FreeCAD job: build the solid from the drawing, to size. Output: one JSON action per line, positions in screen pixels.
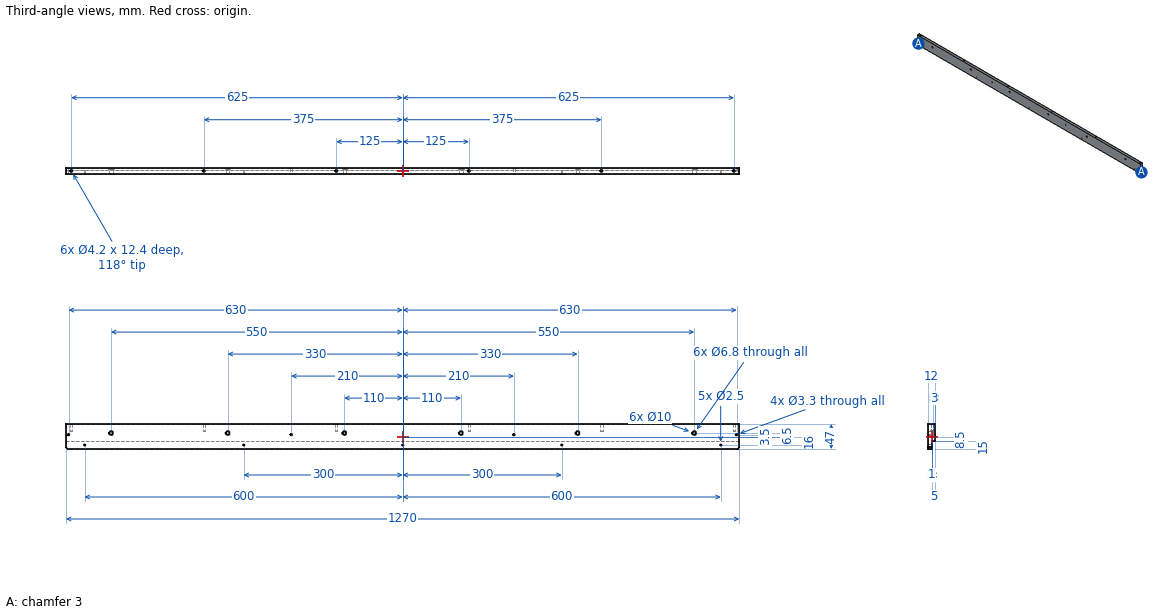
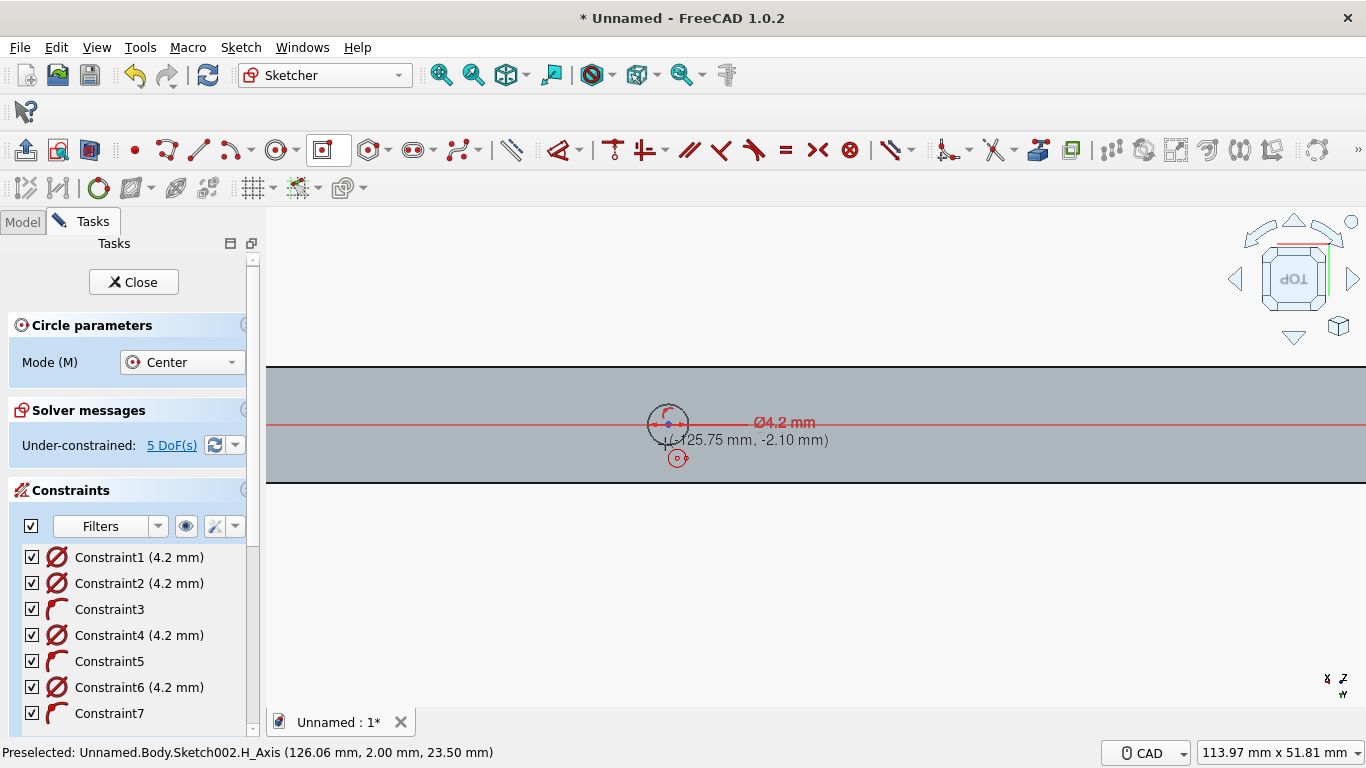
{"action": "scroll", "coordinate": [688, 459], "scroll_direction": "down", "scroll_amount": 15}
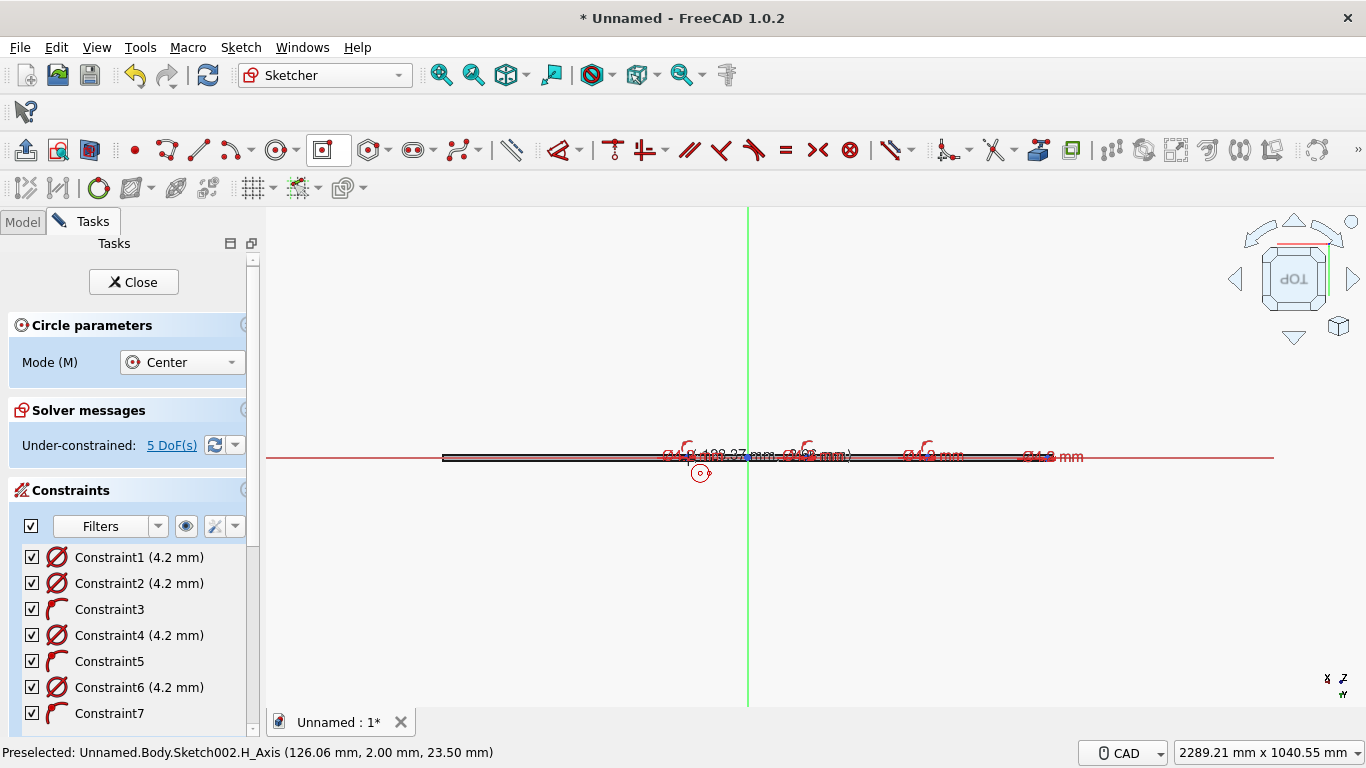
{"action": "scroll", "coordinate": [567, 458], "scroll_direction": "up", "scroll_amount": 16}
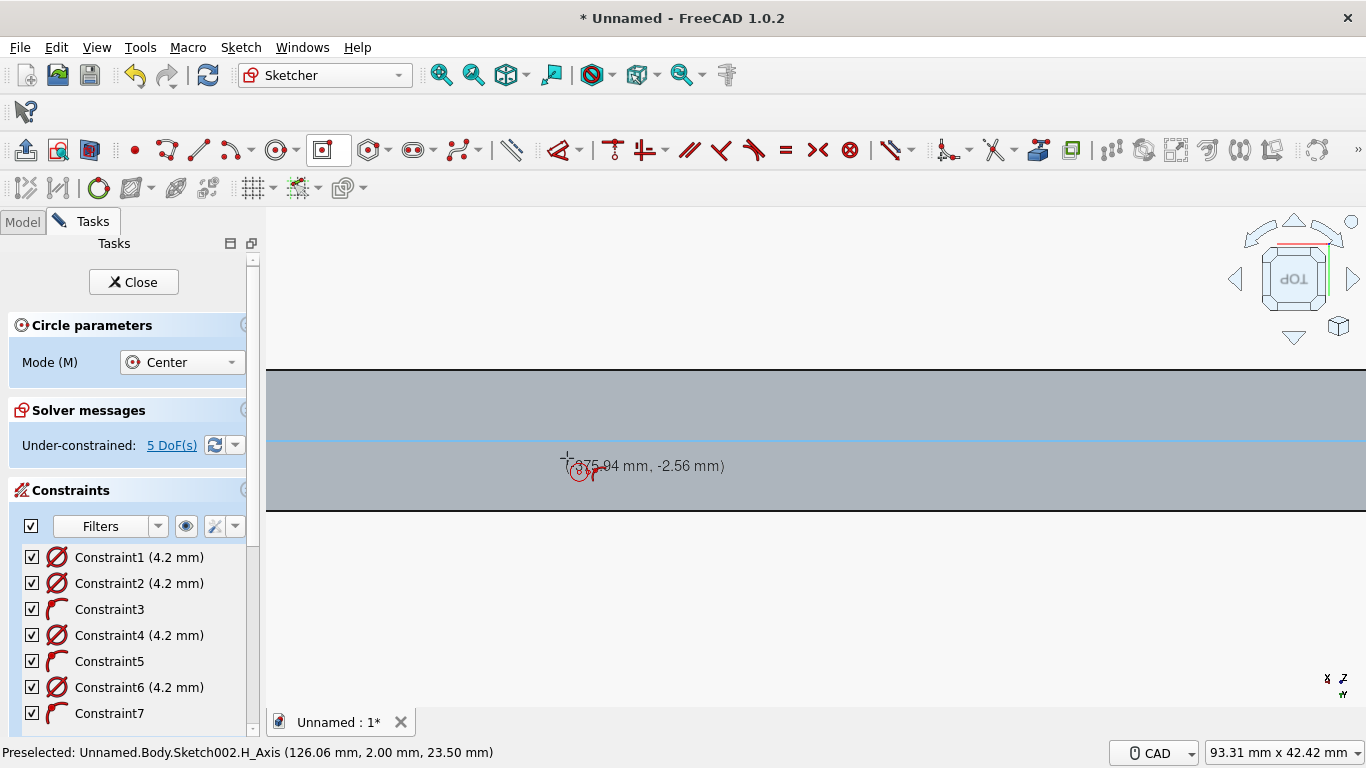
{"action": "scroll", "coordinate": [525, 458], "scroll_direction": "down", "scroll_amount": 15}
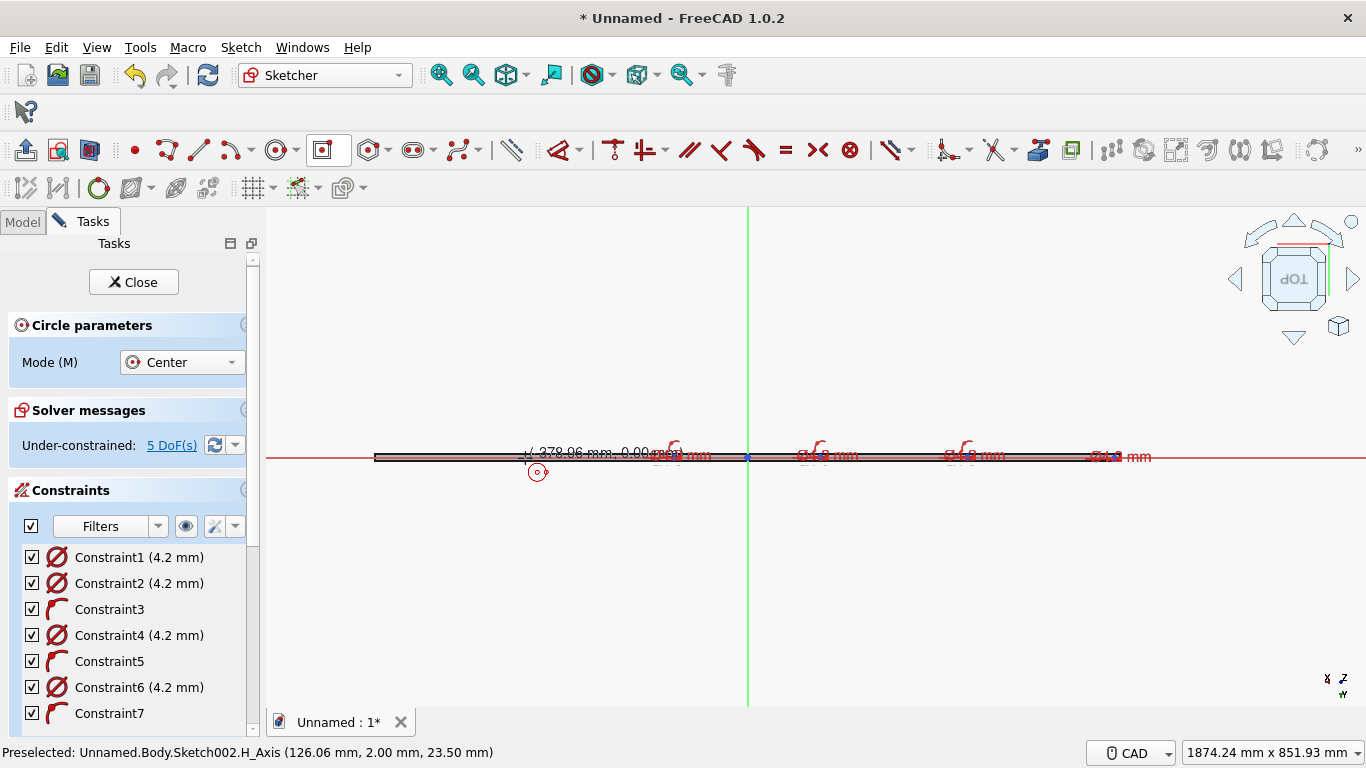
{"action": "left_click", "coordinate": [528, 458]}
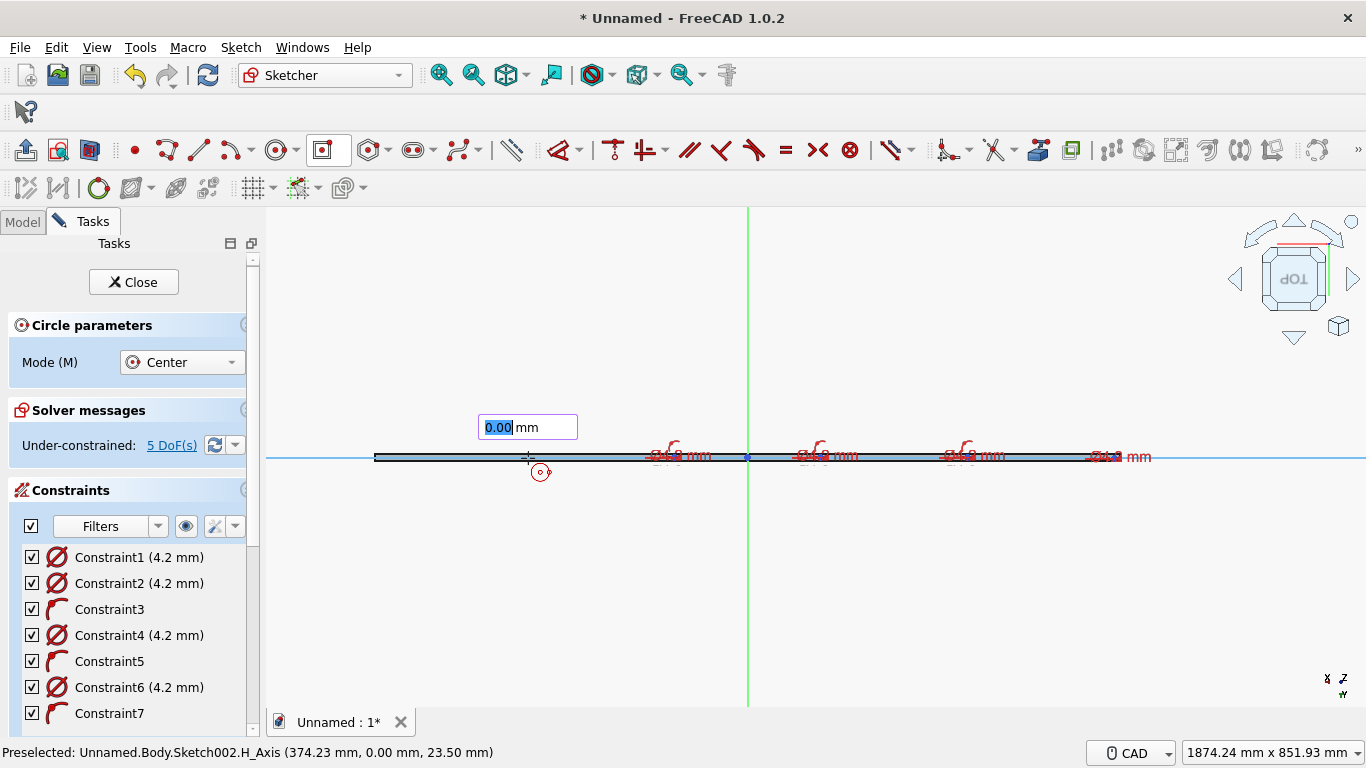
{"action": "scroll", "coordinate": [527, 459], "scroll_direction": "up", "scroll_amount": 14}
{"action": "mouse_move", "coordinate": [525, 447]}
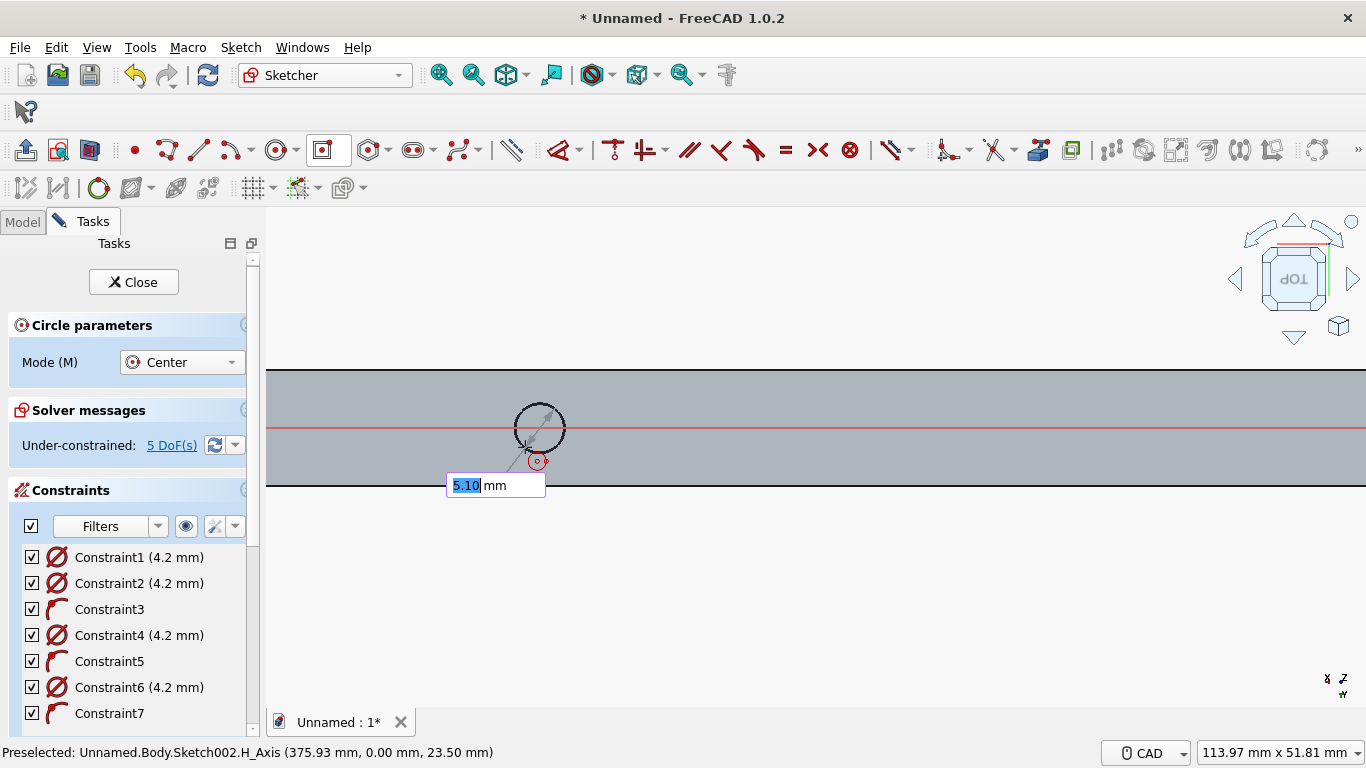
{"action": "type", "text": "4.2"}
{"action": "key", "text": "Return"}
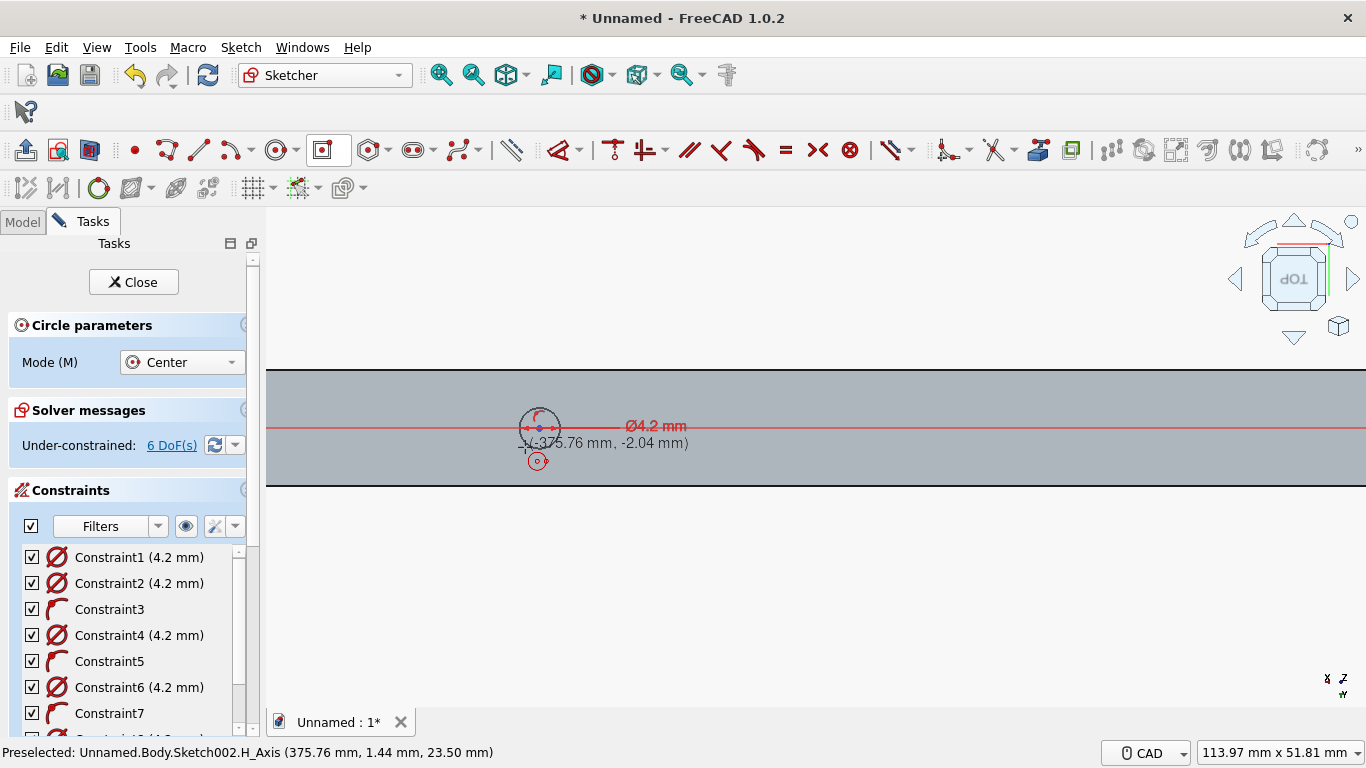
{"action": "scroll", "coordinate": [569, 459], "scroll_direction": "down", "scroll_amount": 15}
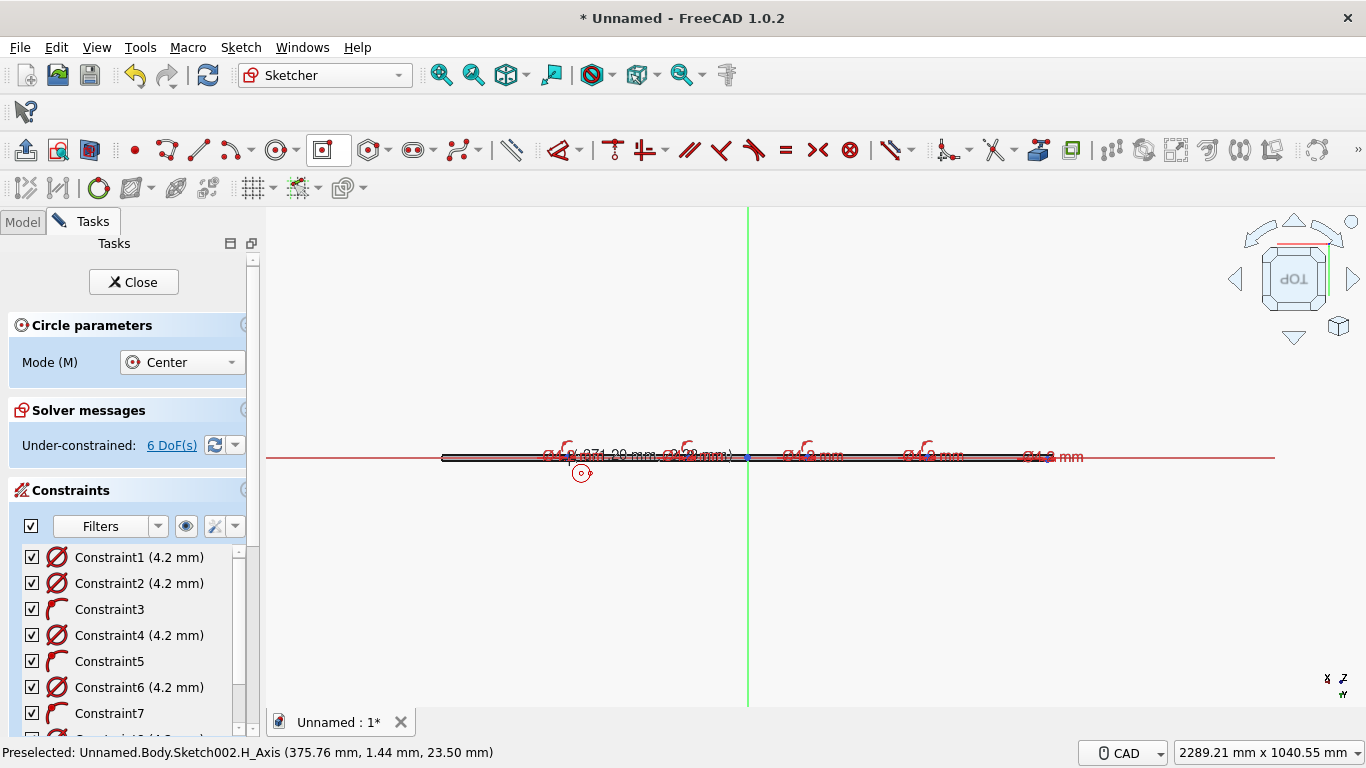
{"action": "scroll", "coordinate": [447, 458], "scroll_direction": "up", "scroll_amount": 16}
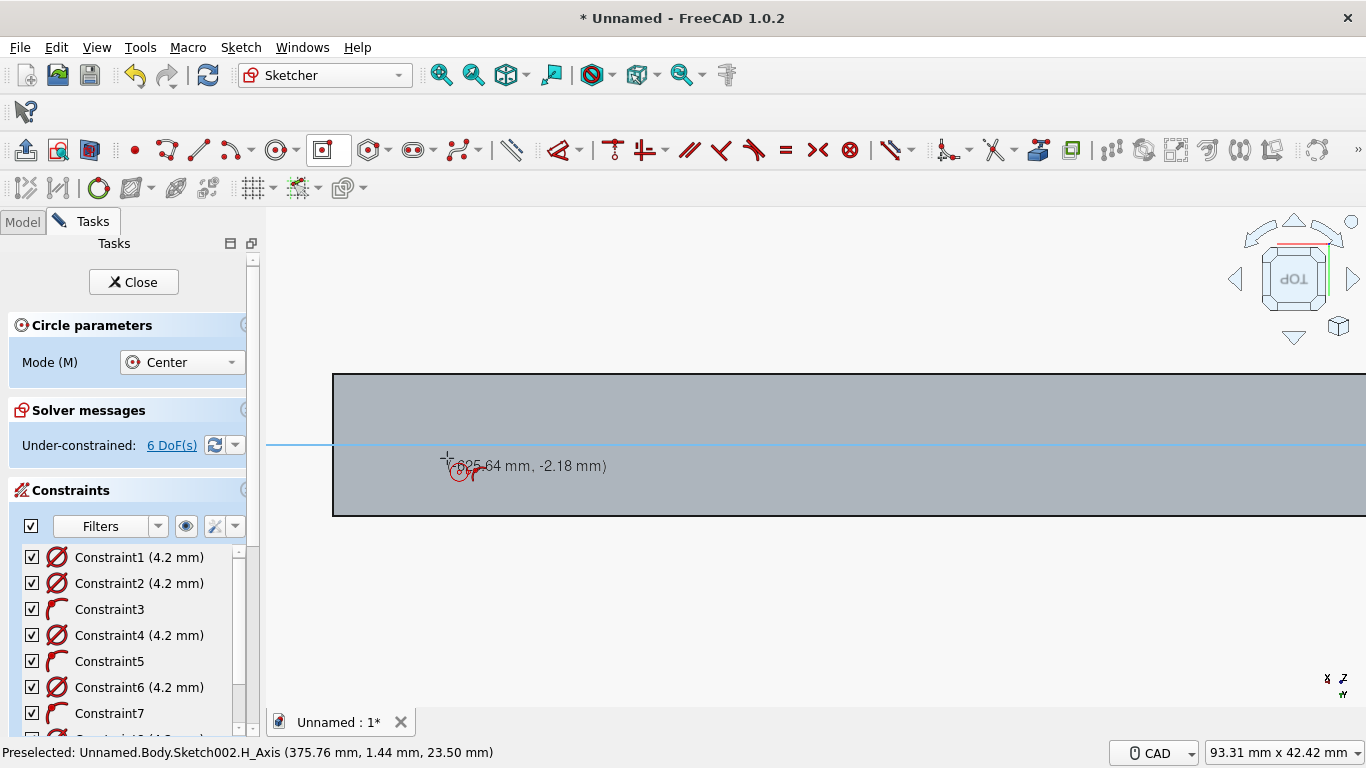
{"action": "scroll", "coordinate": [377, 458], "scroll_direction": "down", "scroll_amount": 15}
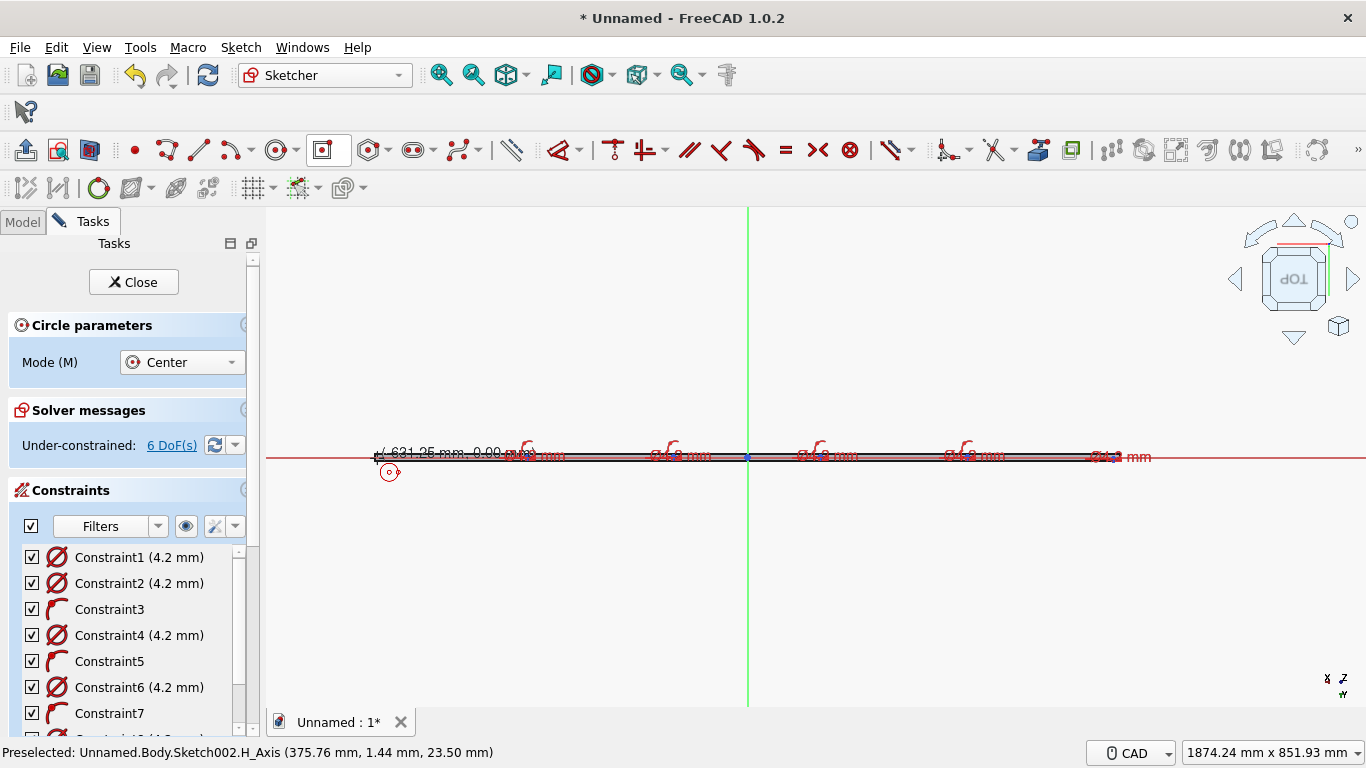
{"action": "left_click", "coordinate": [381, 458]}